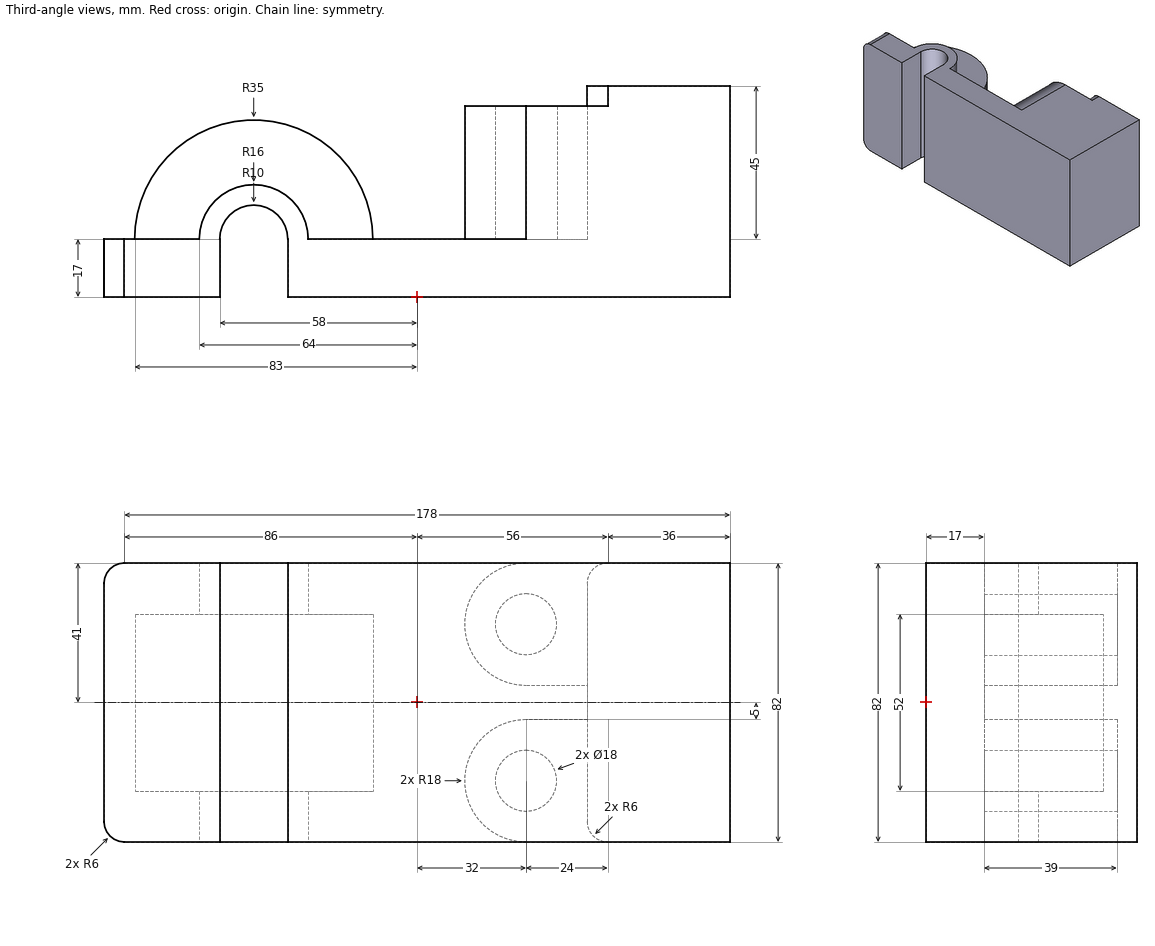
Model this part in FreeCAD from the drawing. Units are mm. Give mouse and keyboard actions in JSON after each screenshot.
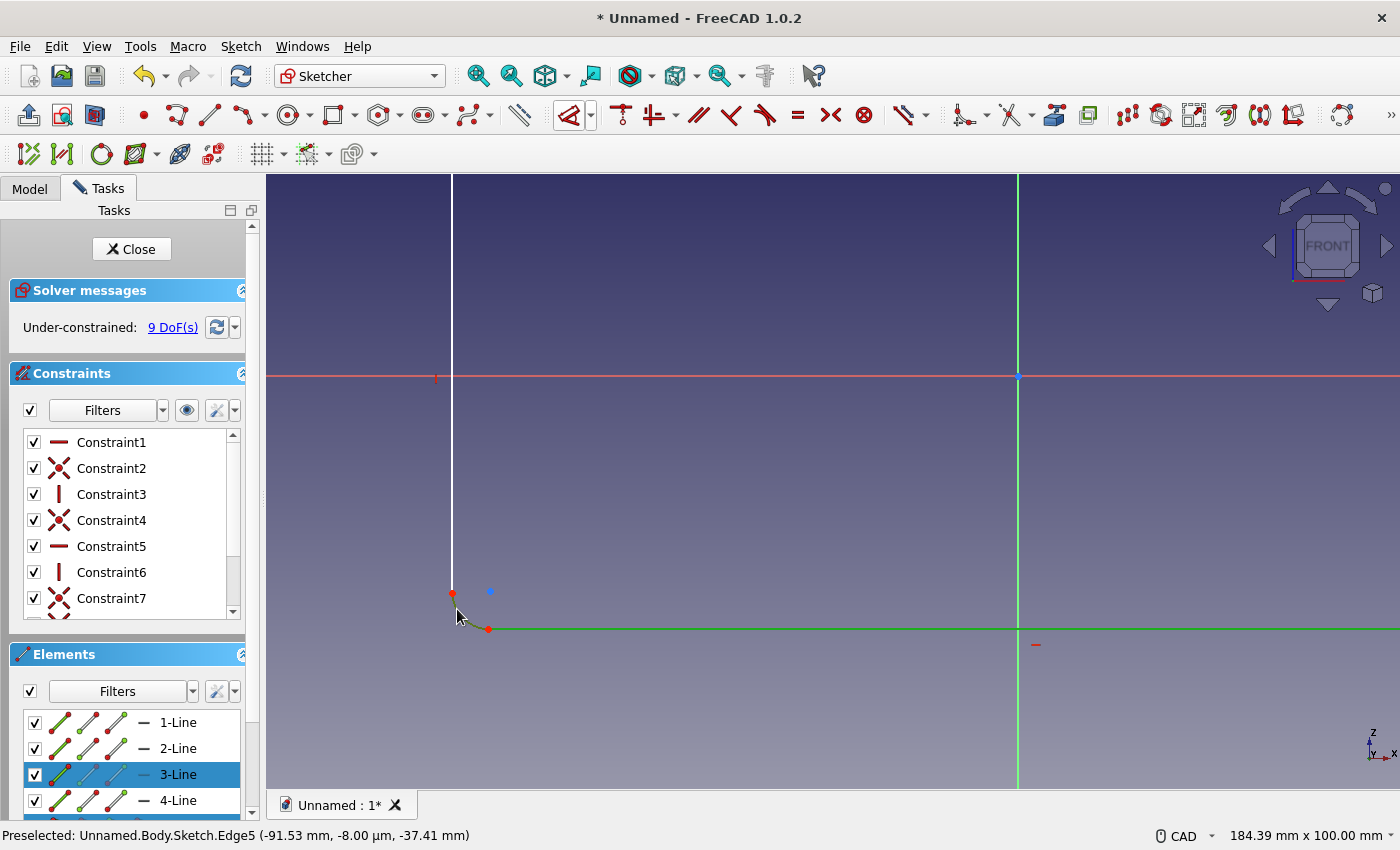
{"action": "left_click", "coordinate": [765, 116]}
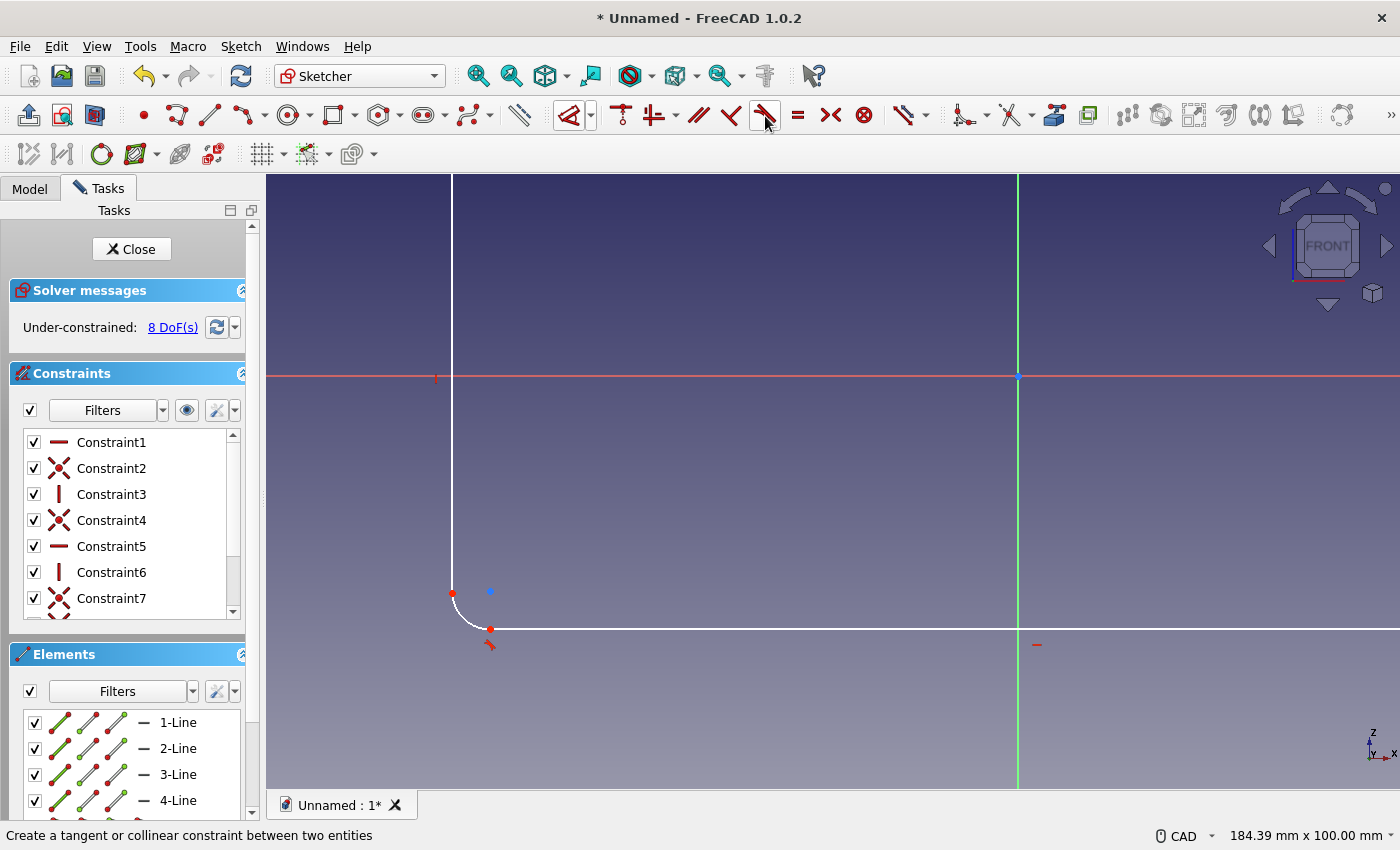
{"action": "left_click", "coordinate": [452, 464]}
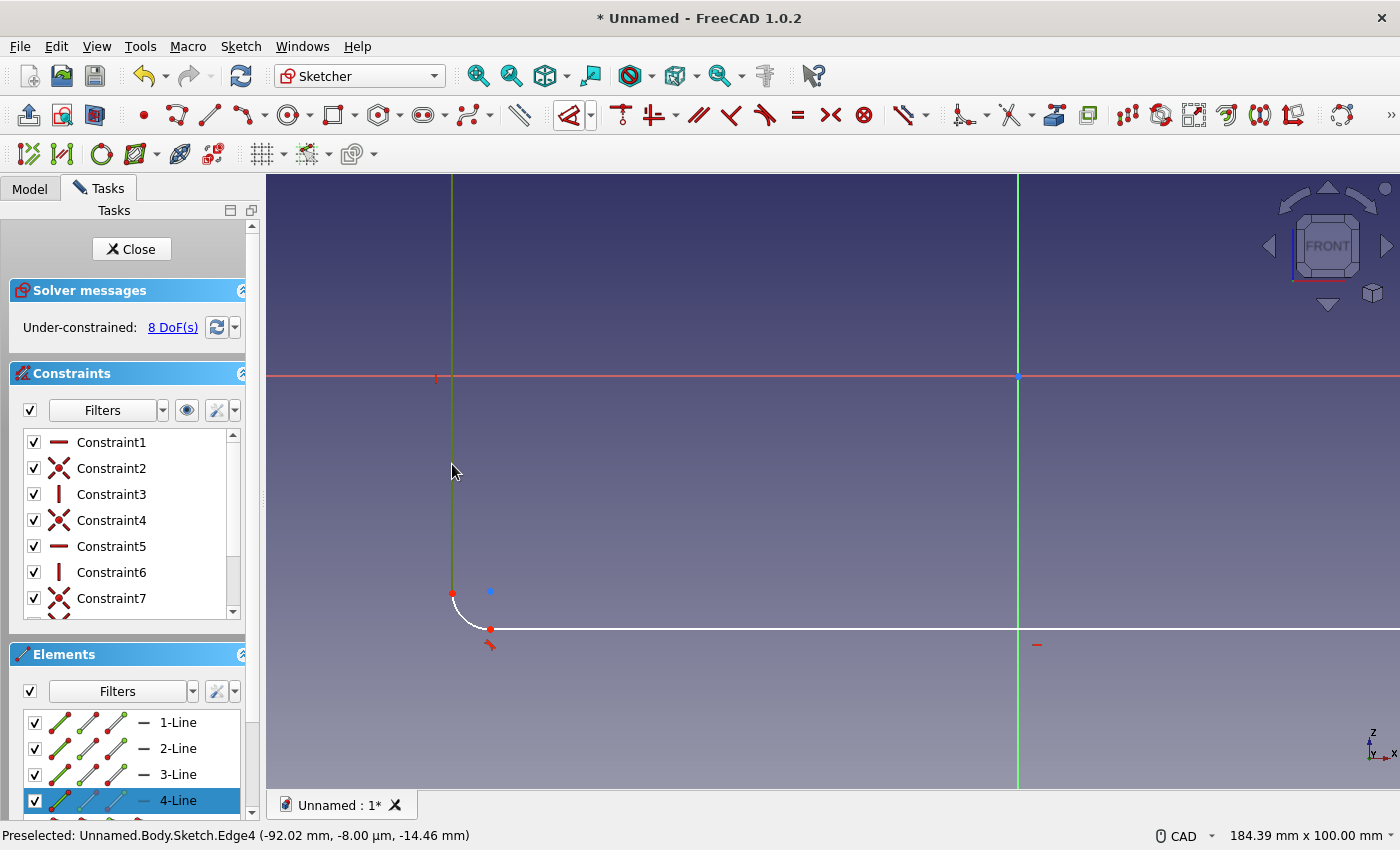
{"action": "left_click", "coordinate": [457, 610]}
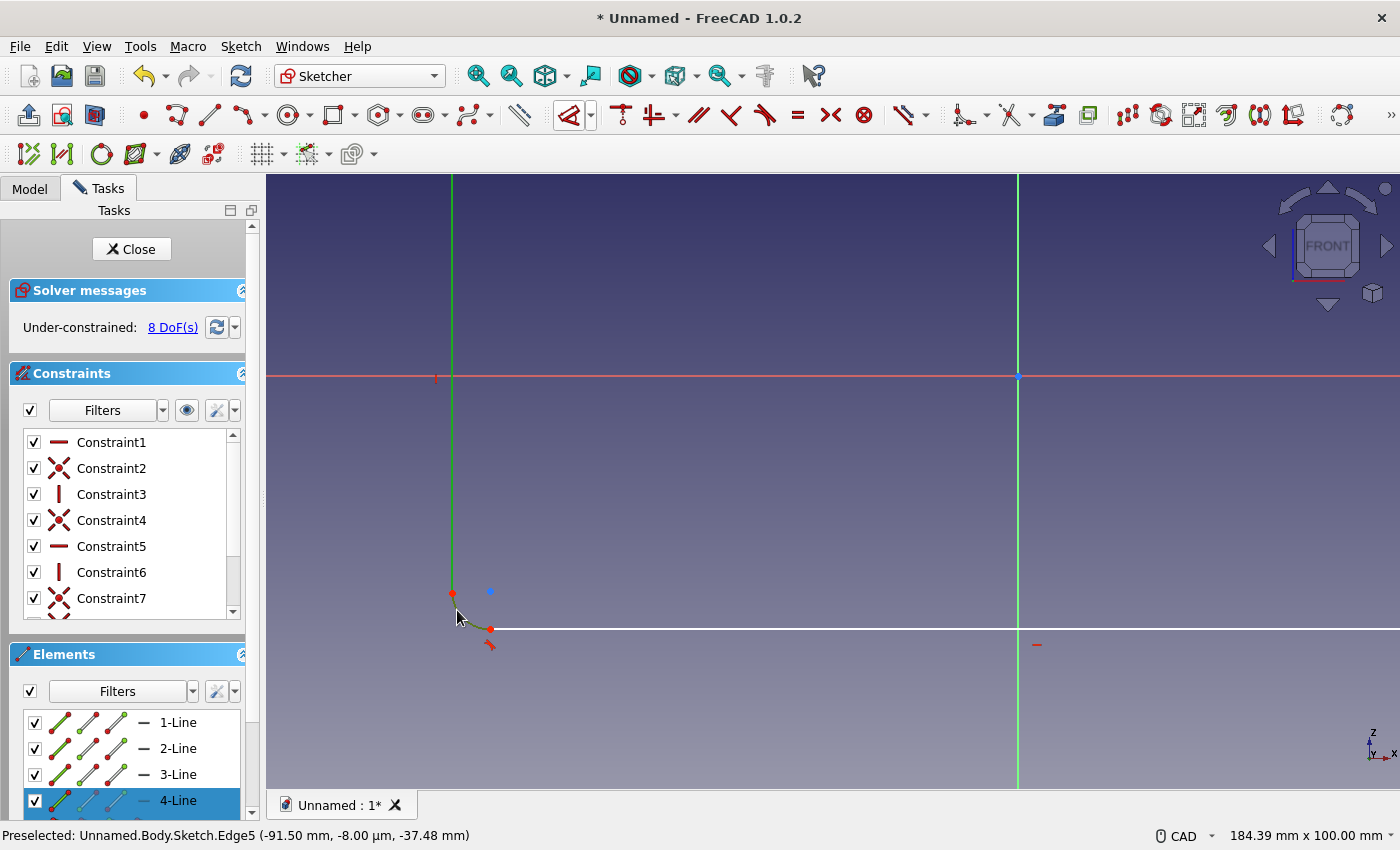
{"action": "left_click", "coordinate": [765, 116]}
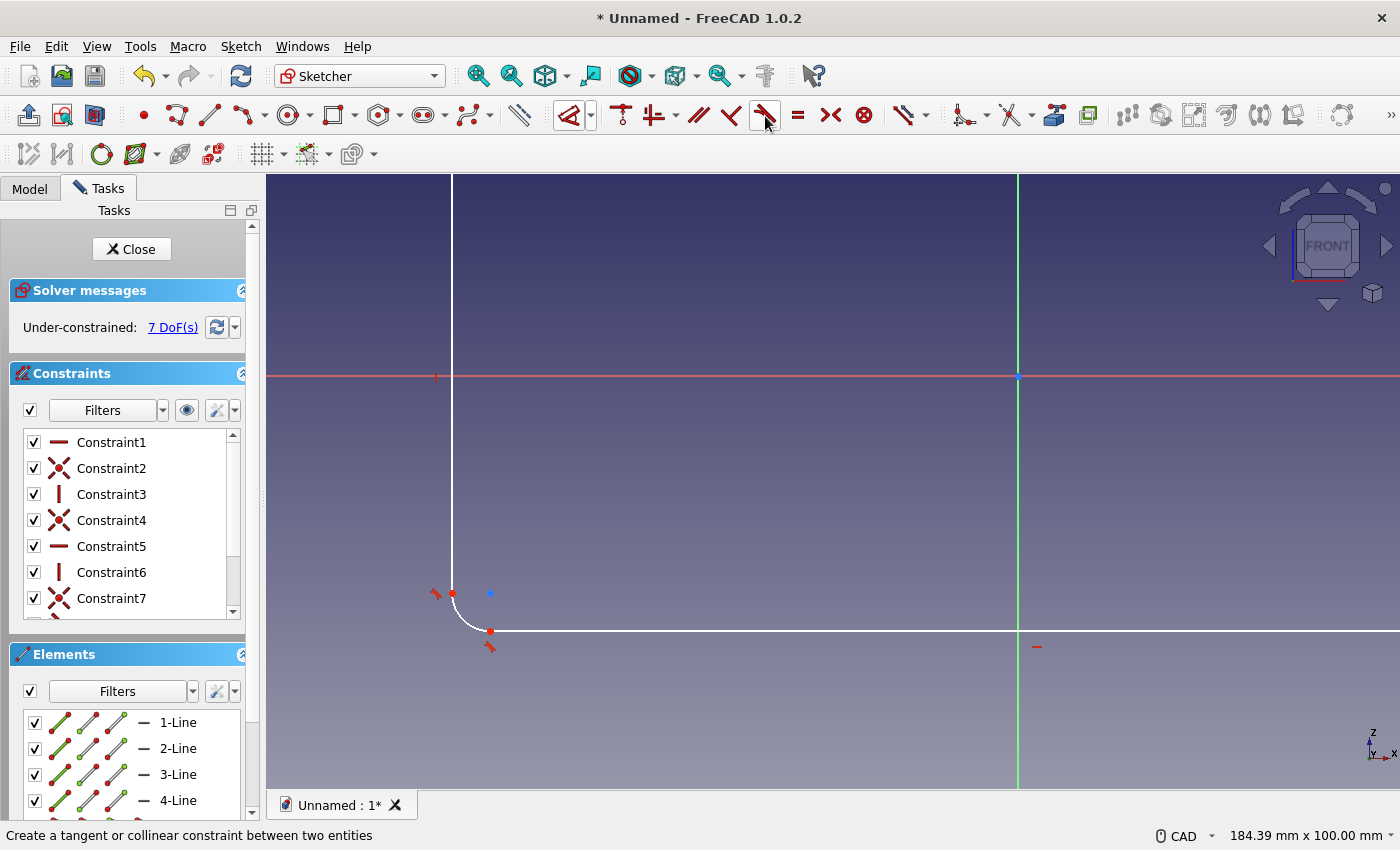
{"action": "left_click", "coordinate": [452, 464]}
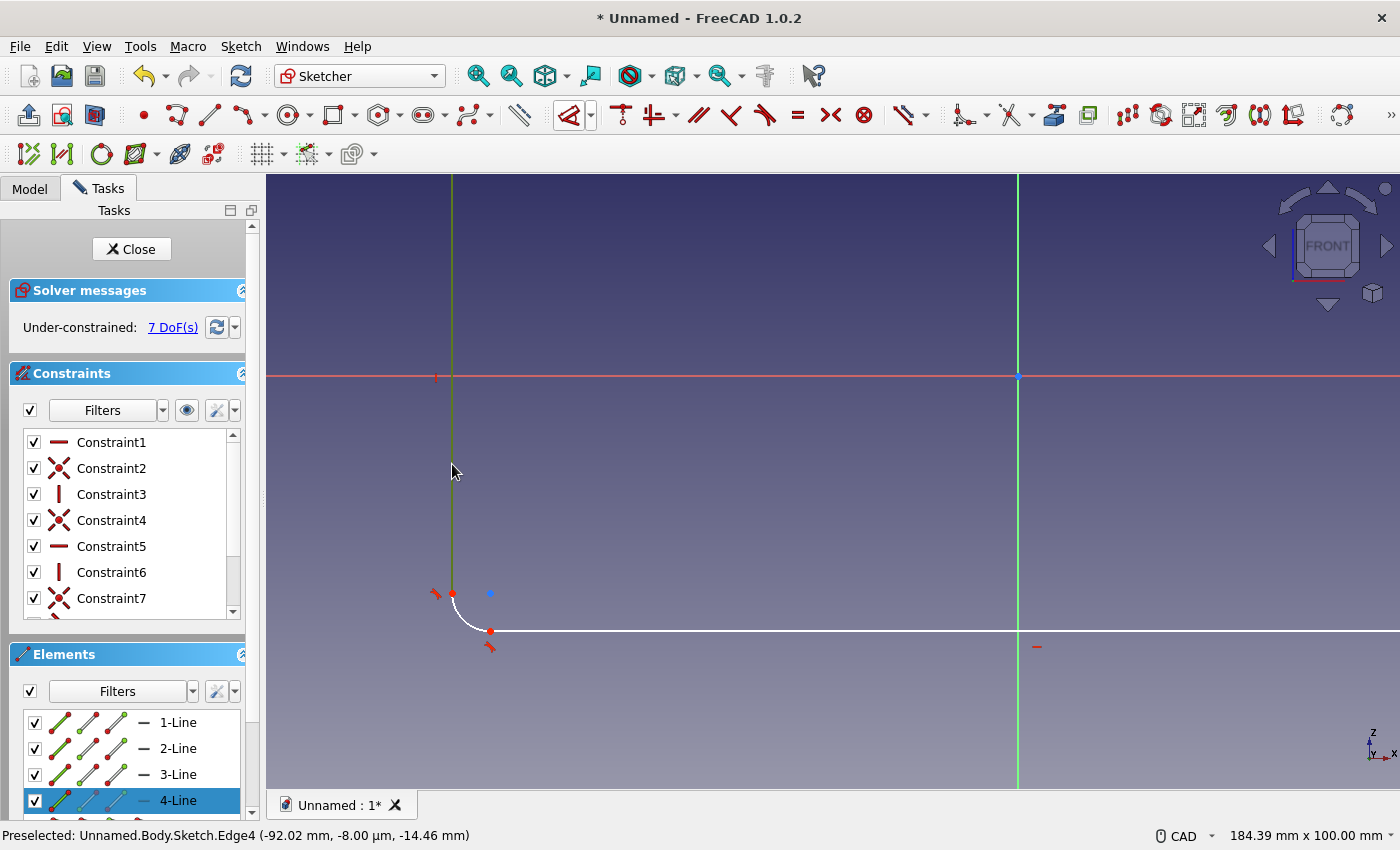
{"action": "scroll", "coordinate": [456, 610], "scroll_direction": "down", "scroll_amount": 3}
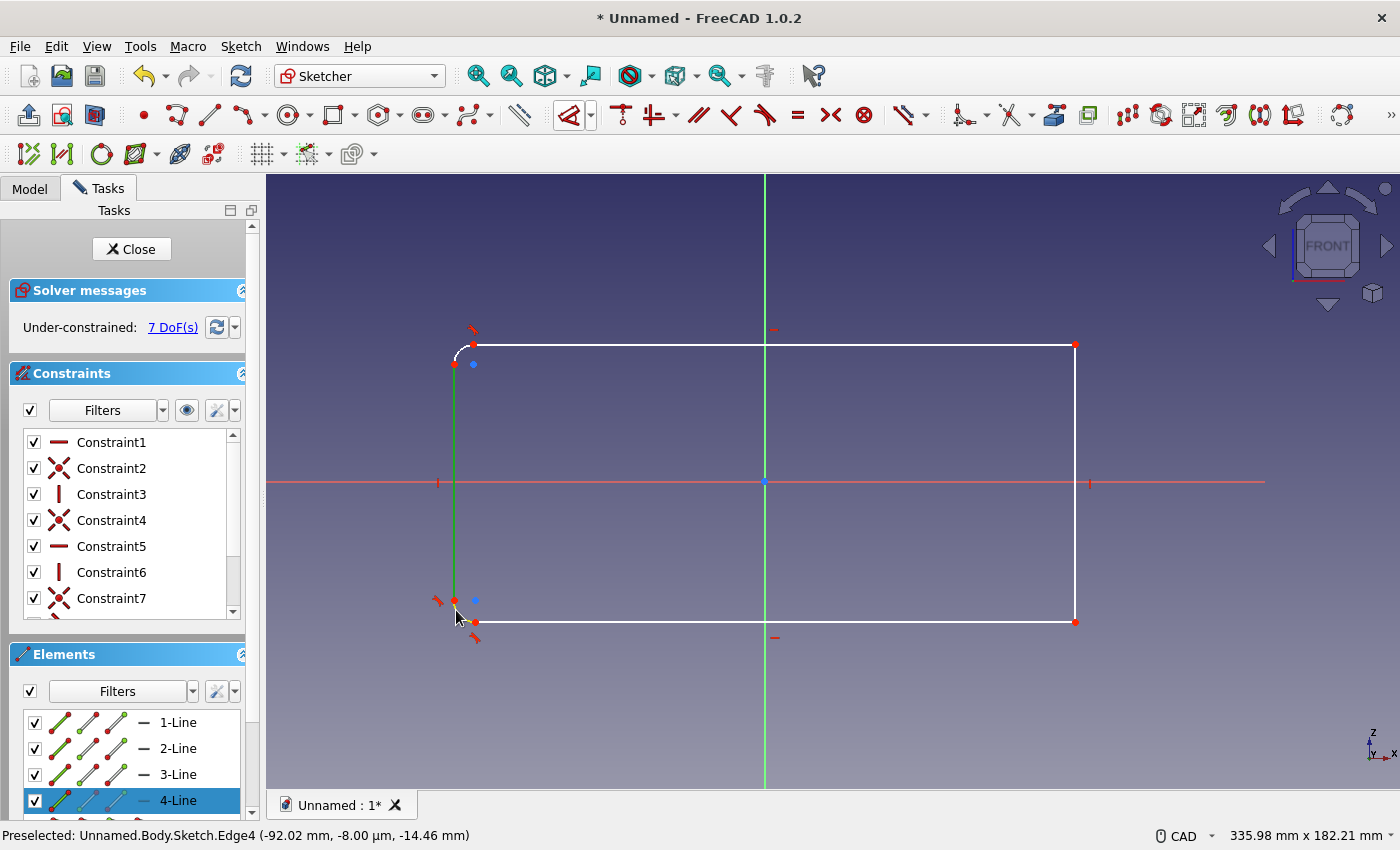
{"action": "scroll", "coordinate": [465, 347], "scroll_direction": "up", "scroll_amount": 2}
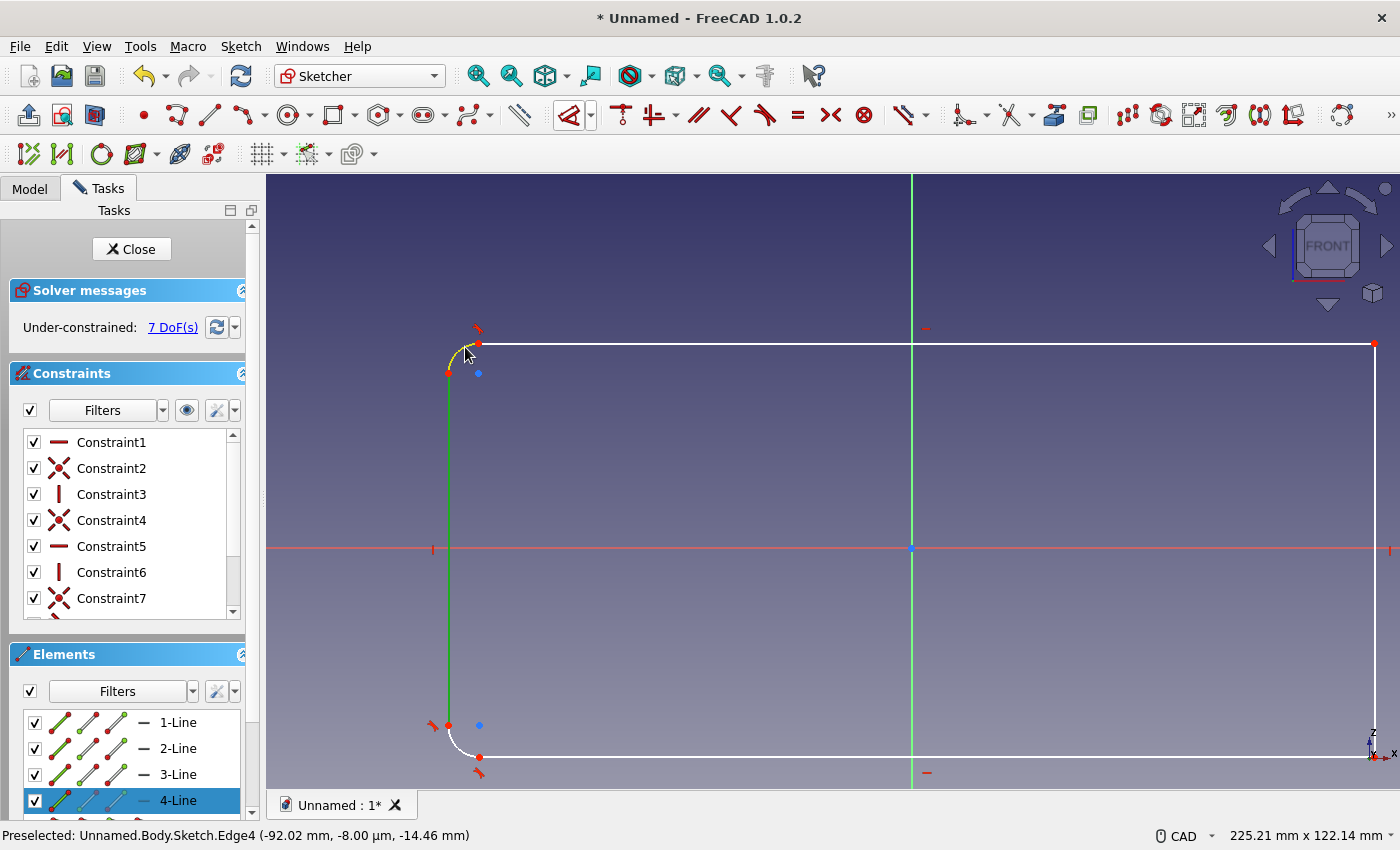
{"action": "left_click", "coordinate": [465, 347]}